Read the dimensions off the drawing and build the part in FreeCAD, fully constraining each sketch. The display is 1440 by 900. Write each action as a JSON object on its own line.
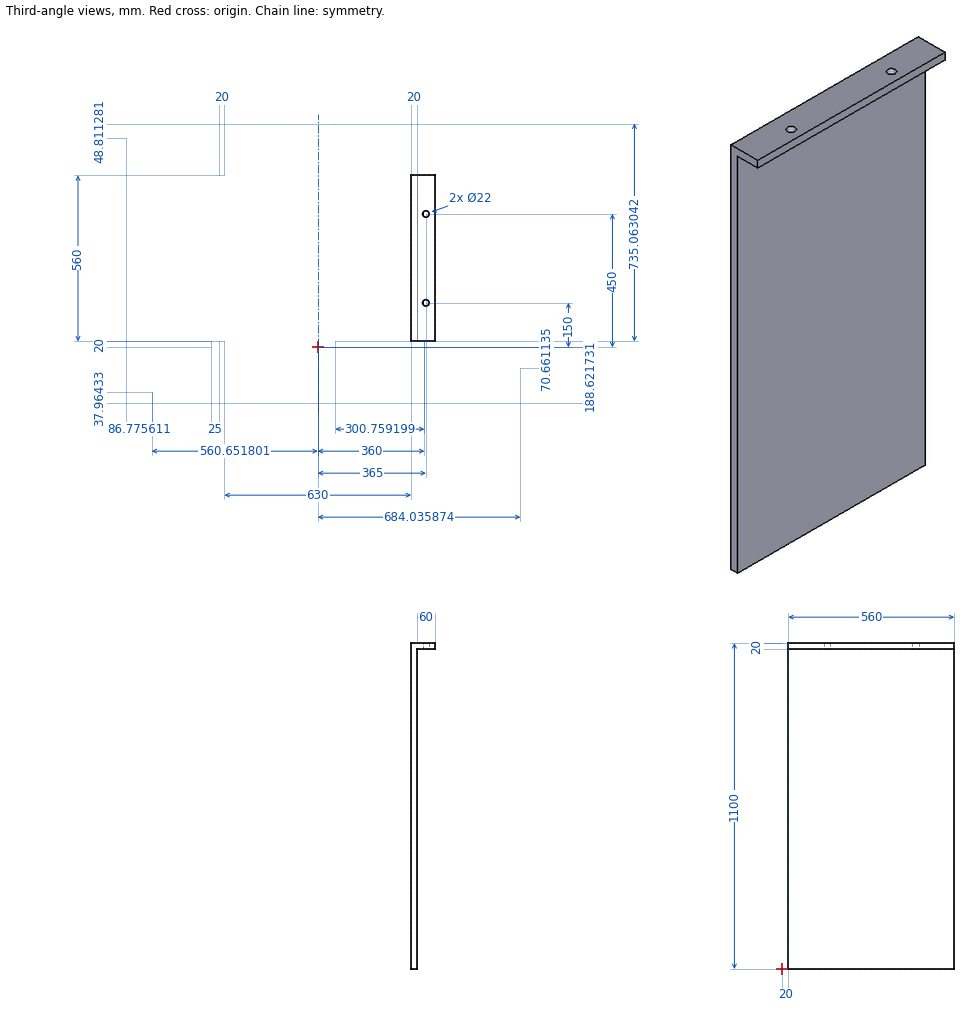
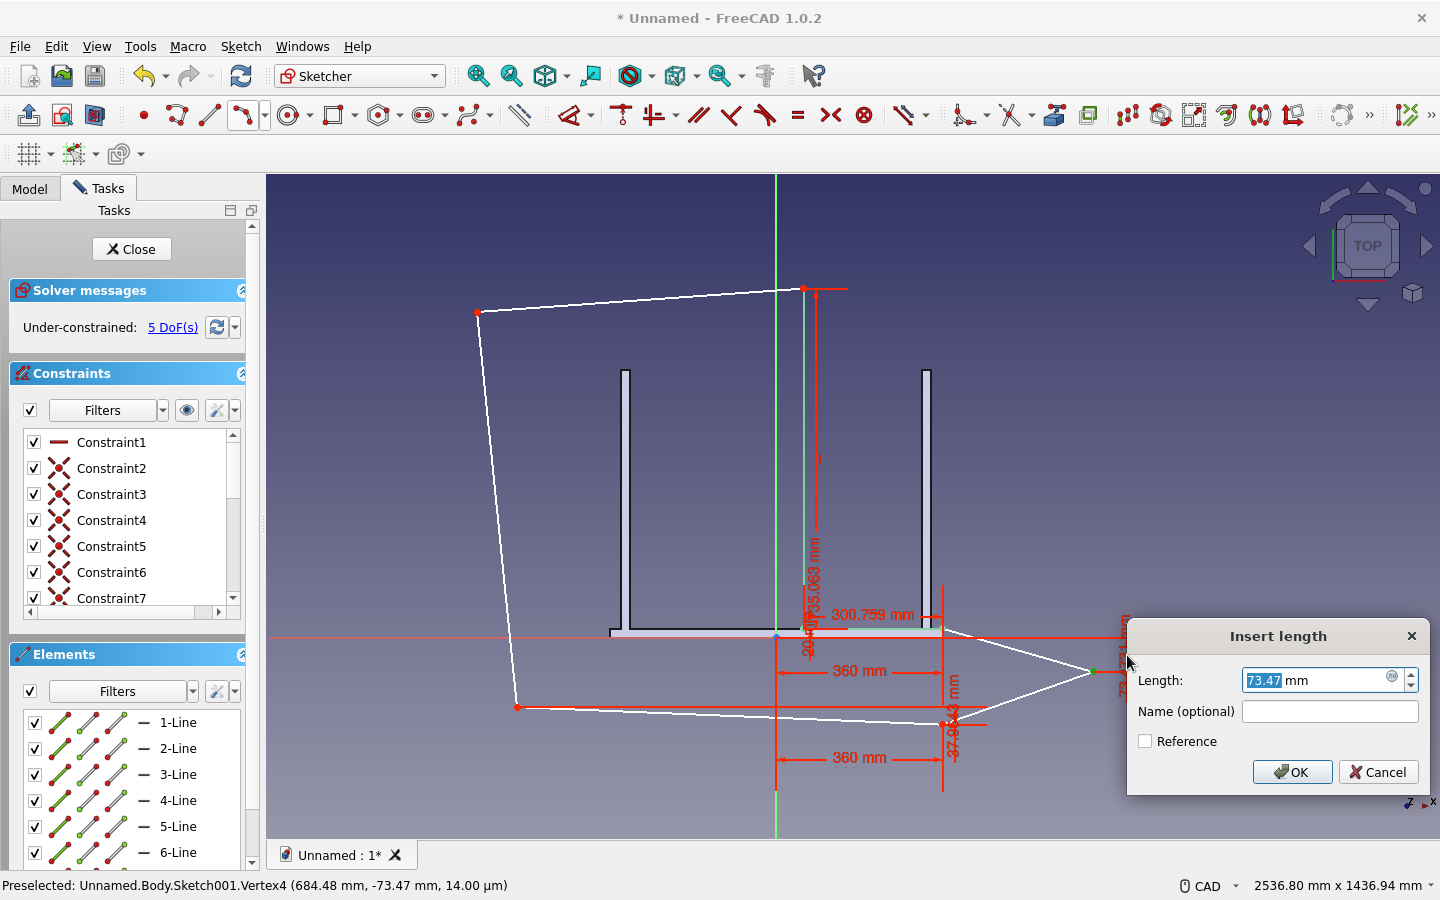
{"action": "type", "text": "70.661135"}
{"action": "key", "text": "Return"}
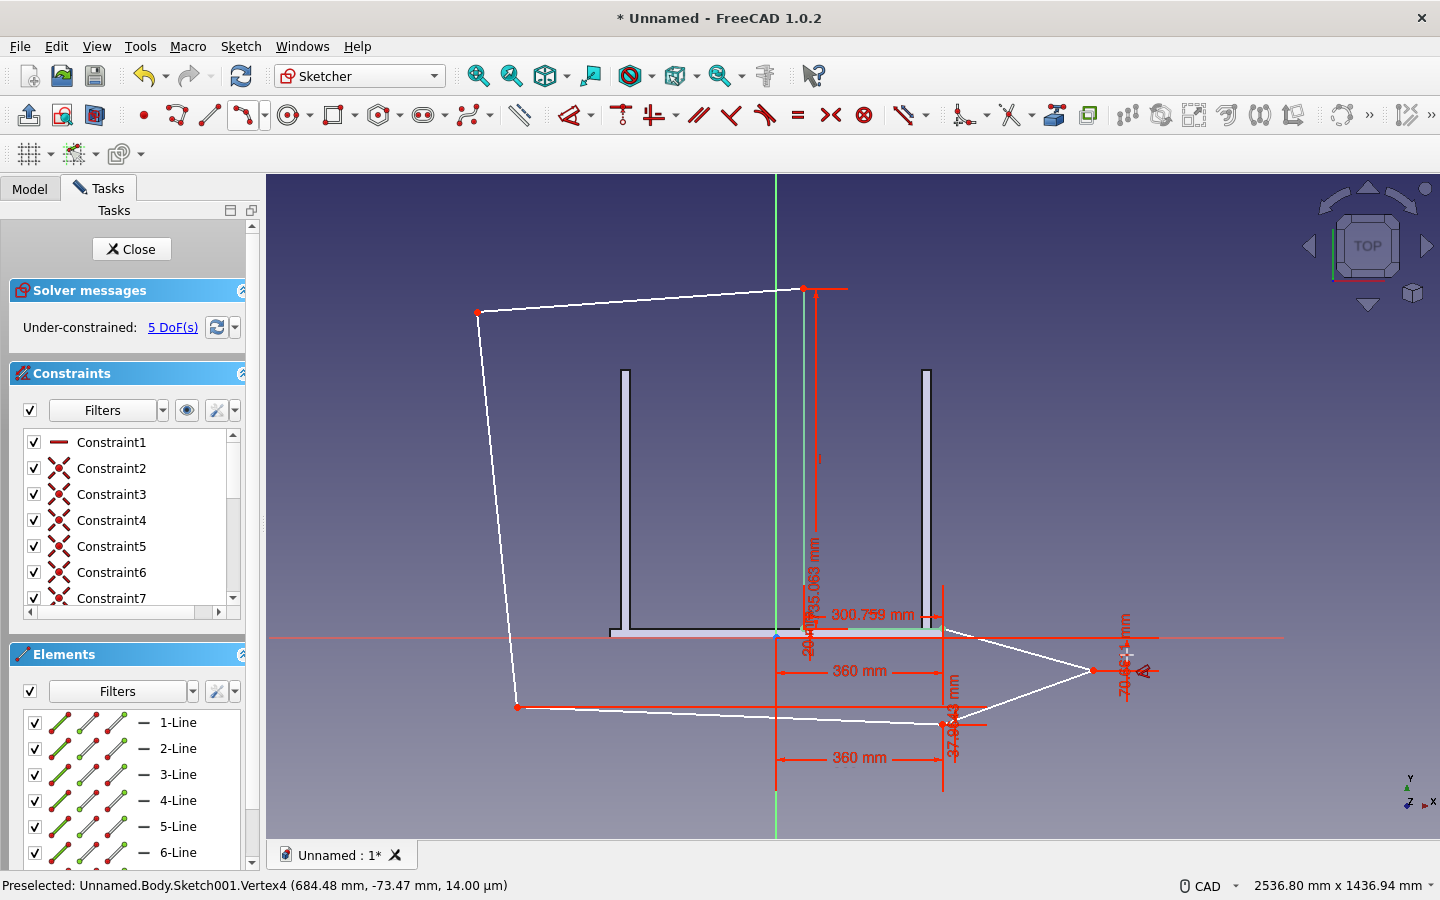
{"action": "left_click", "coordinate": [505, 589]}
{"action": "left_click", "coordinate": [497, 741]}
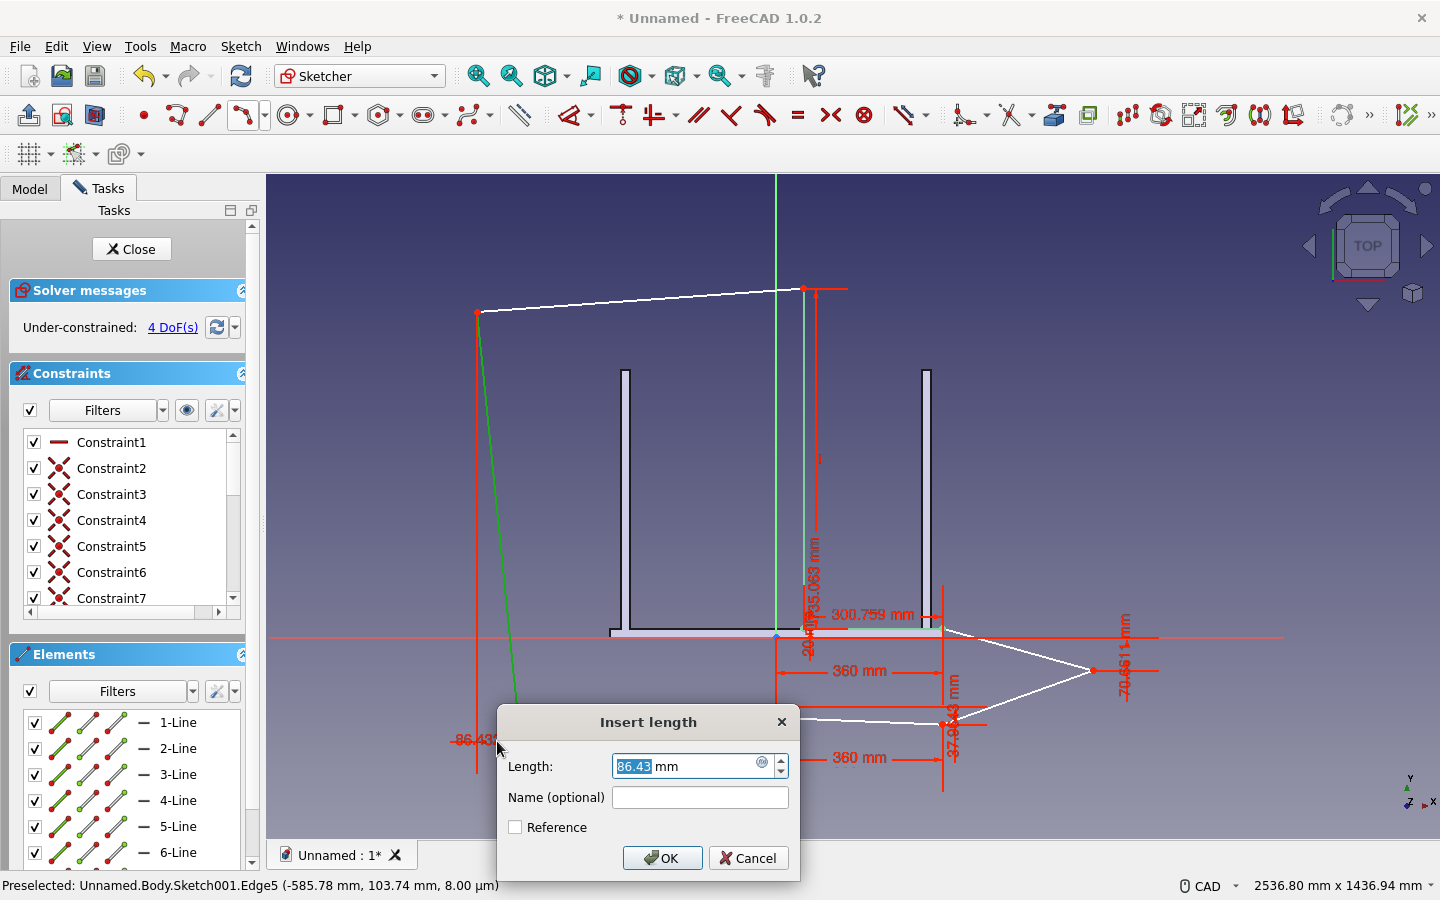
{"action": "type", "text": "86.775611"}
{"action": "key", "text": "Return"}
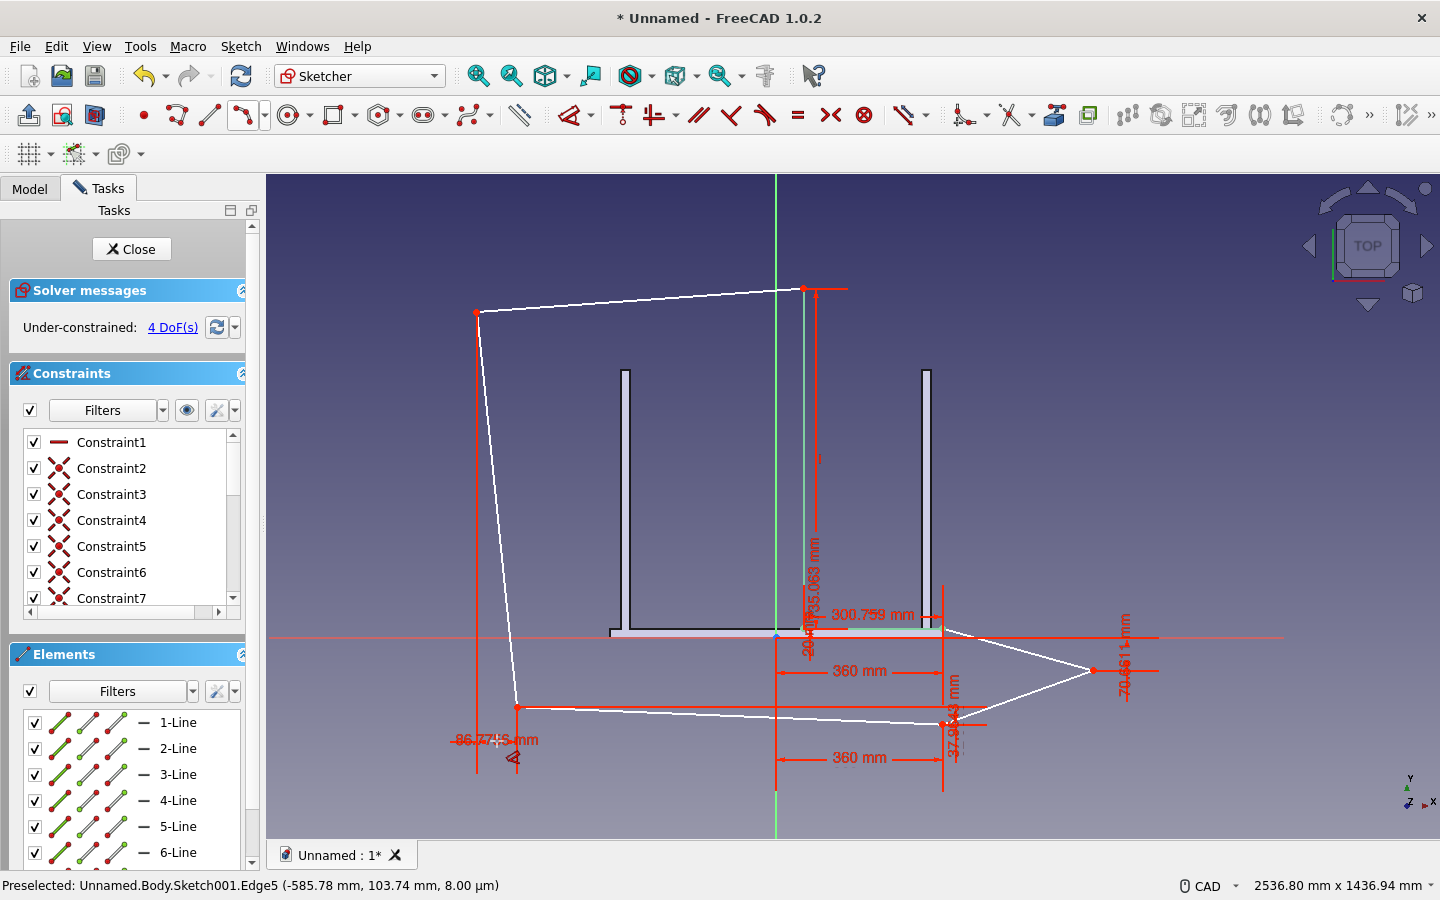
{"action": "scroll", "coordinate": [575, 305], "scroll_direction": "up", "scroll_amount": 3}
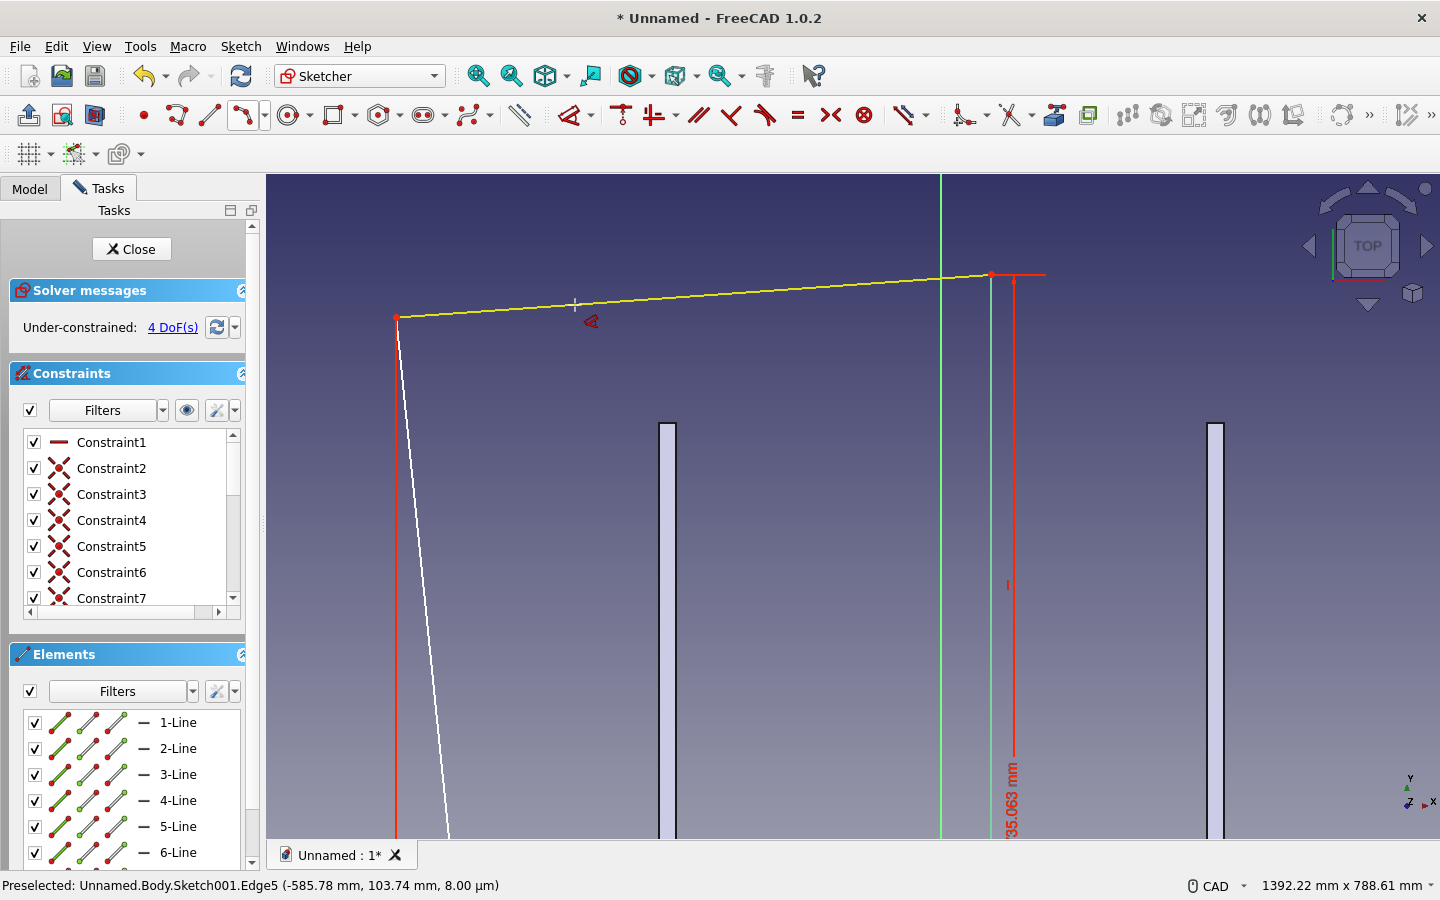
{"action": "left_click", "coordinate": [575, 305]}
{"action": "left_click", "coordinate": [362, 296]}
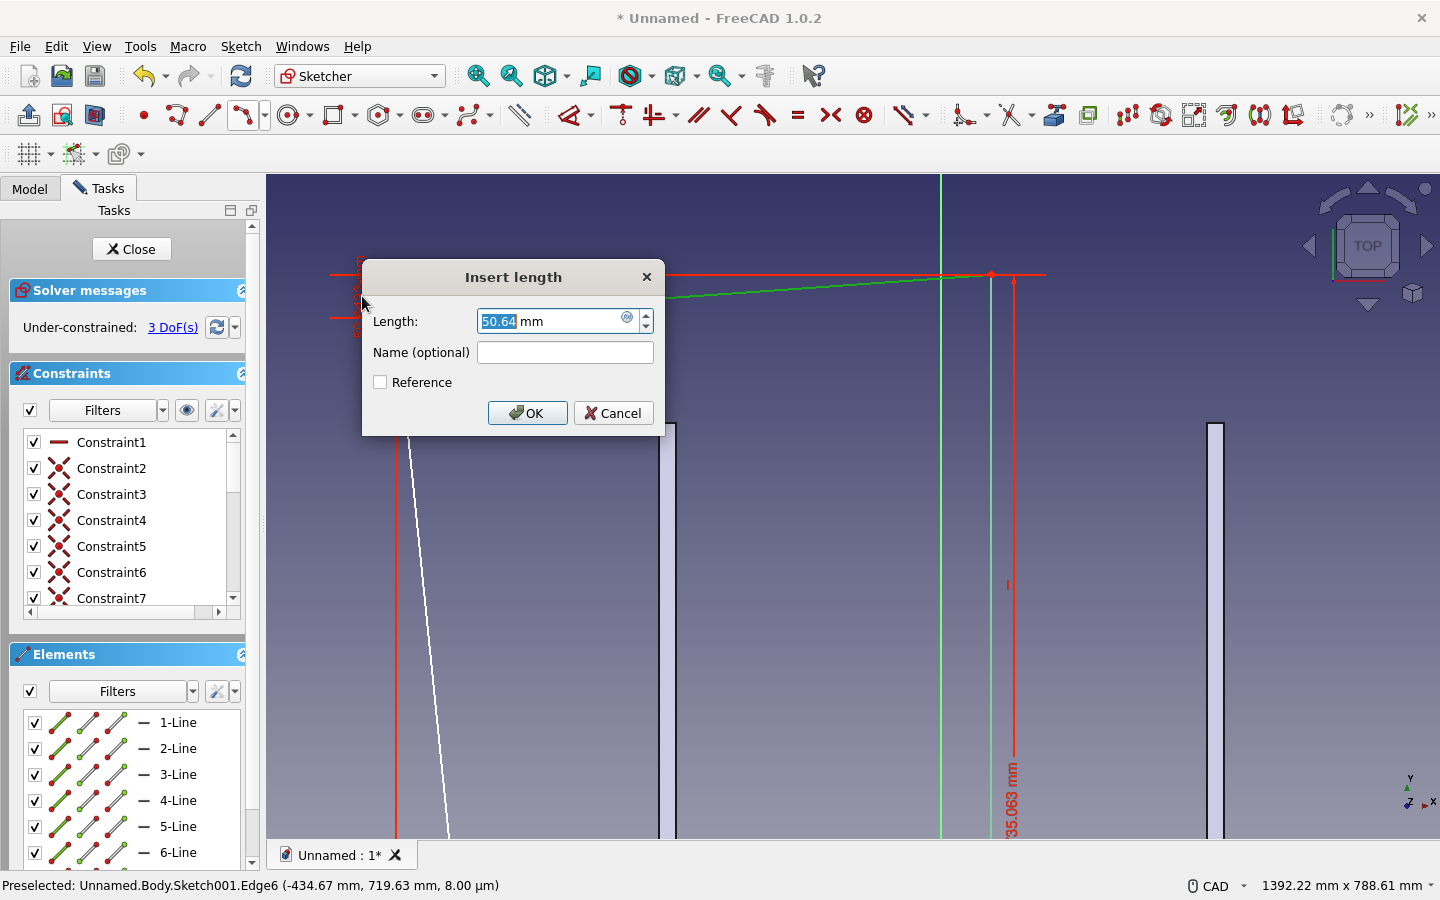
{"action": "type", "text": "48.811281"}
{"action": "key", "text": "Return"}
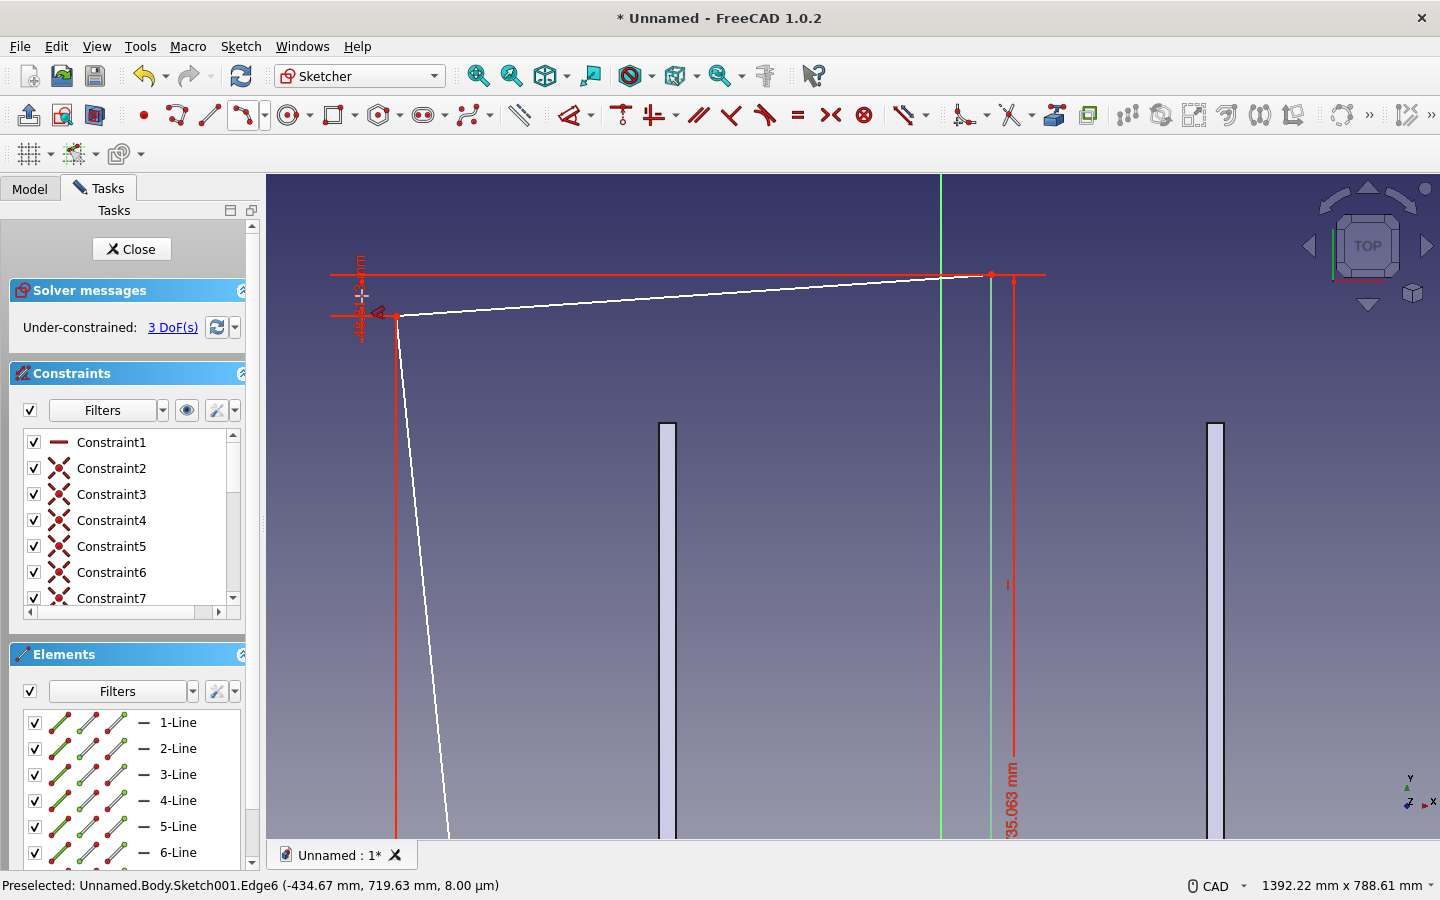
{"action": "scroll", "coordinate": [575, 304], "scroll_direction": "down", "scroll_amount": 3}